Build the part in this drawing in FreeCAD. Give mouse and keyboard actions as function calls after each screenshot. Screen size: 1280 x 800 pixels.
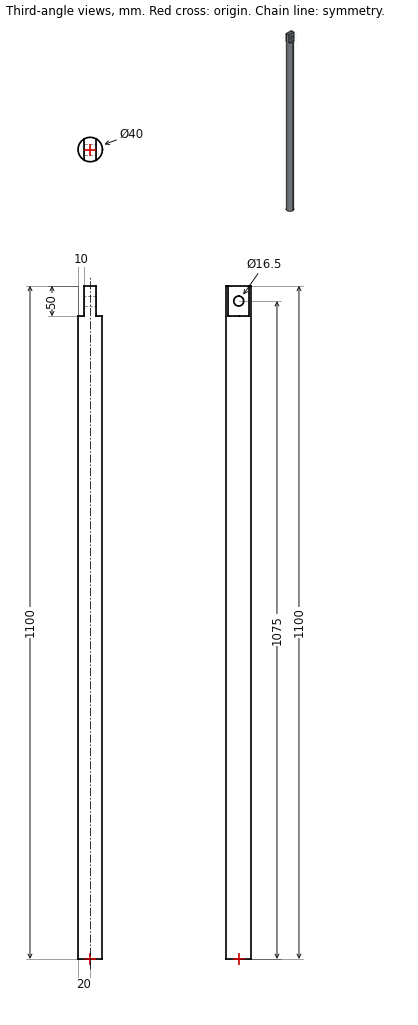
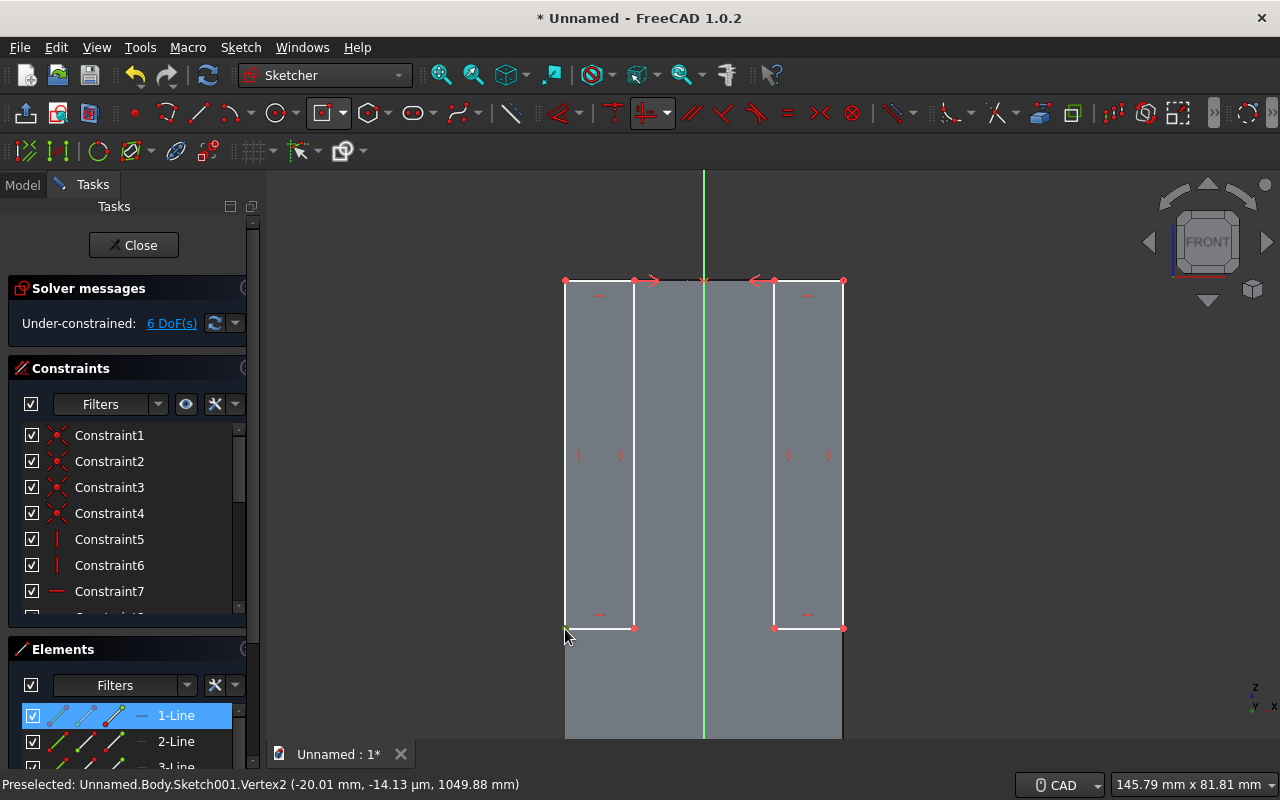
click(843, 629)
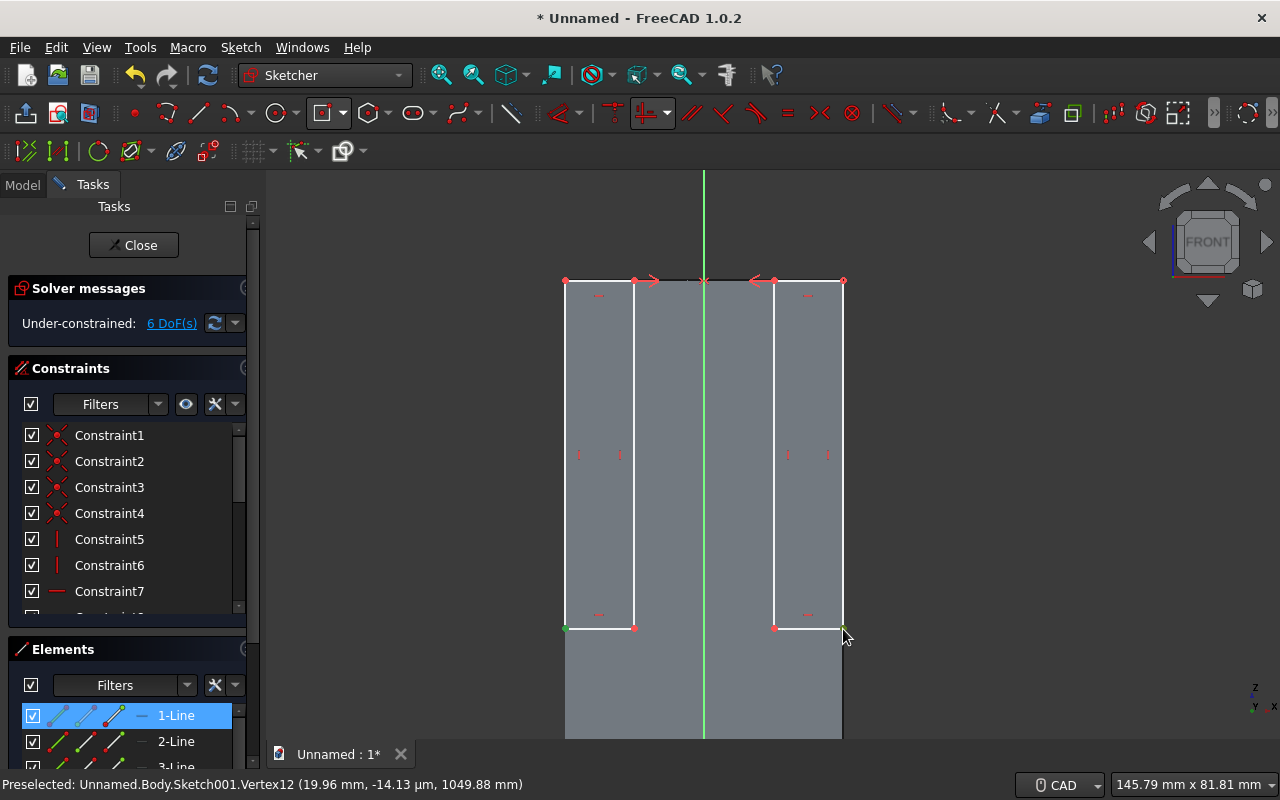
click(704, 674)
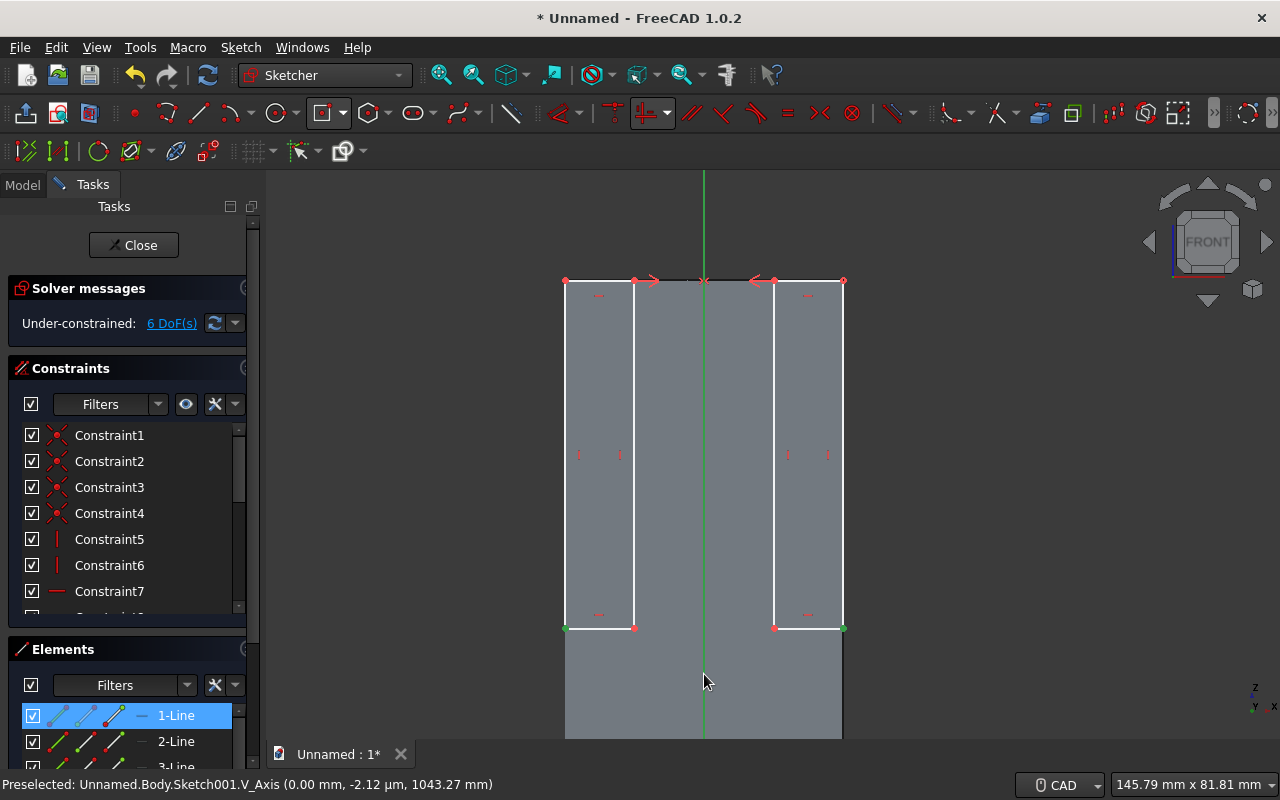
click(820, 114)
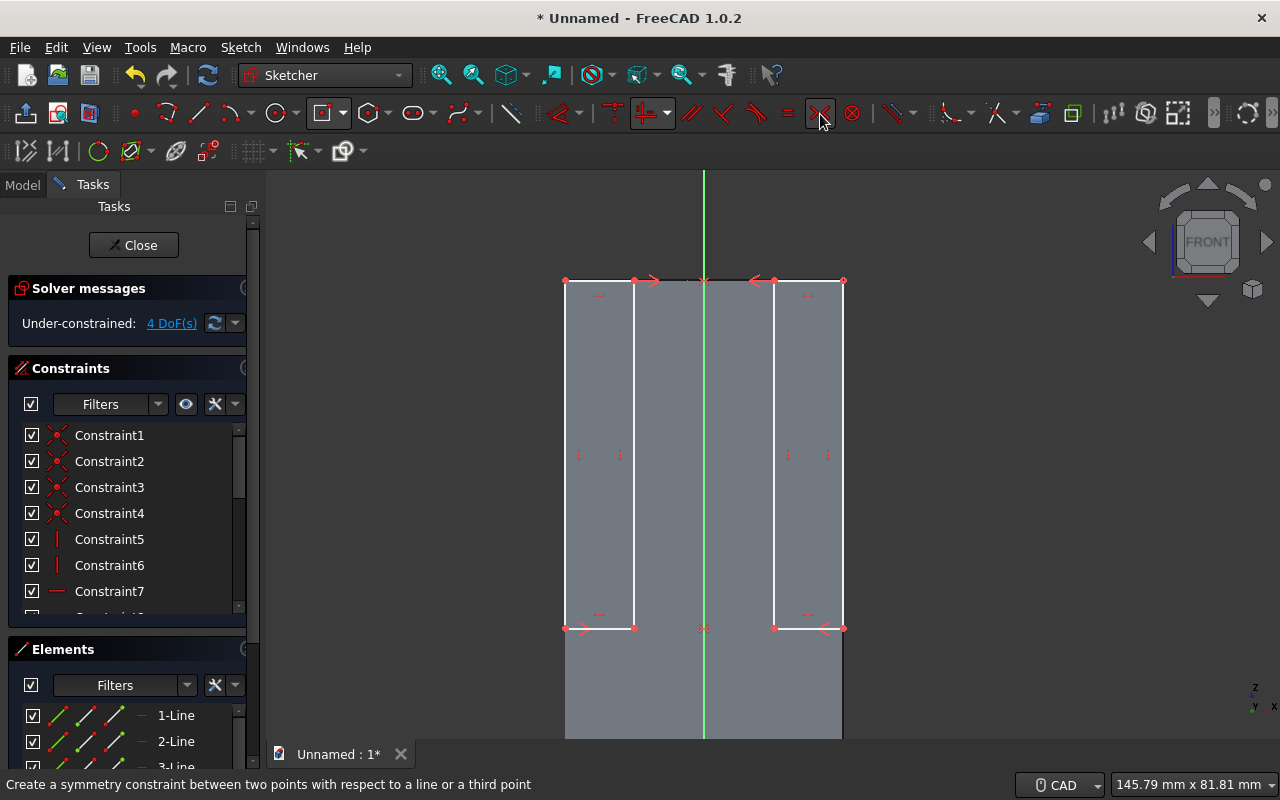
click(558, 114)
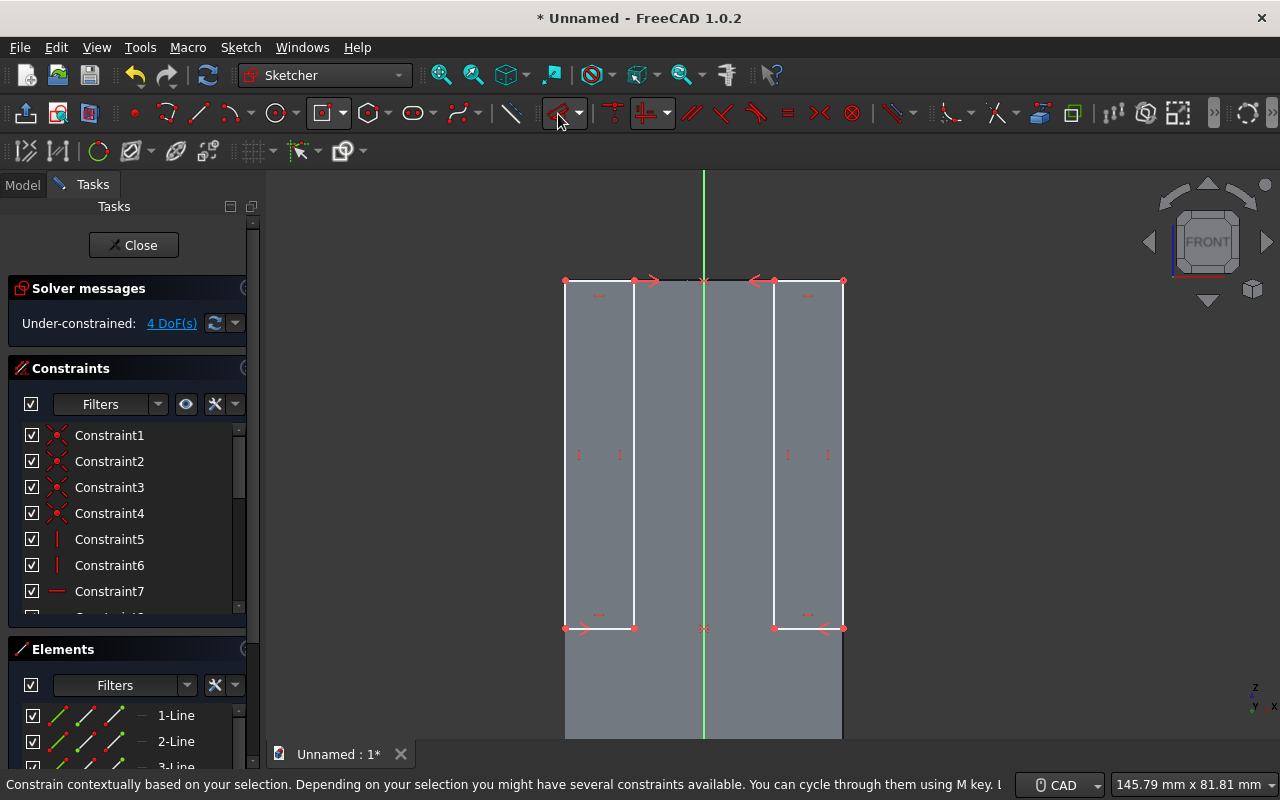
click(565, 385)
click(531, 455)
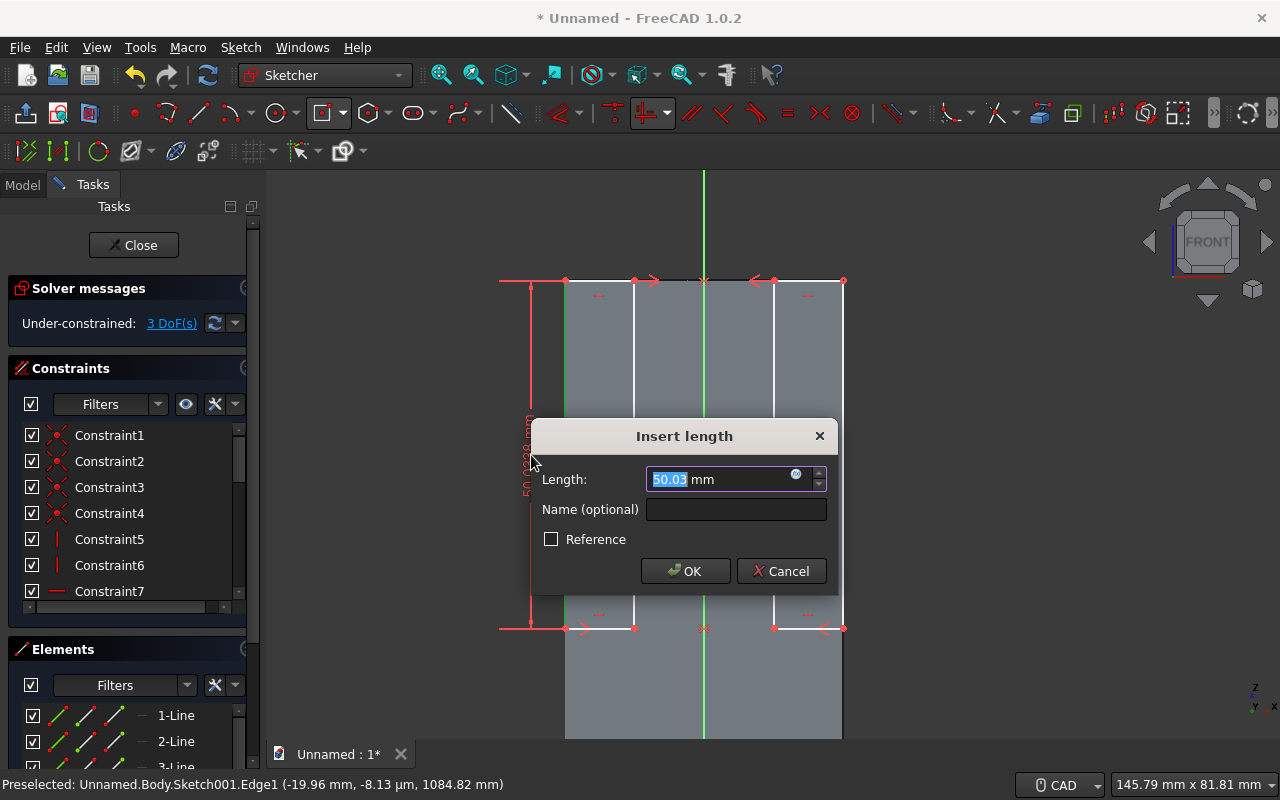
text(50)
key(Return)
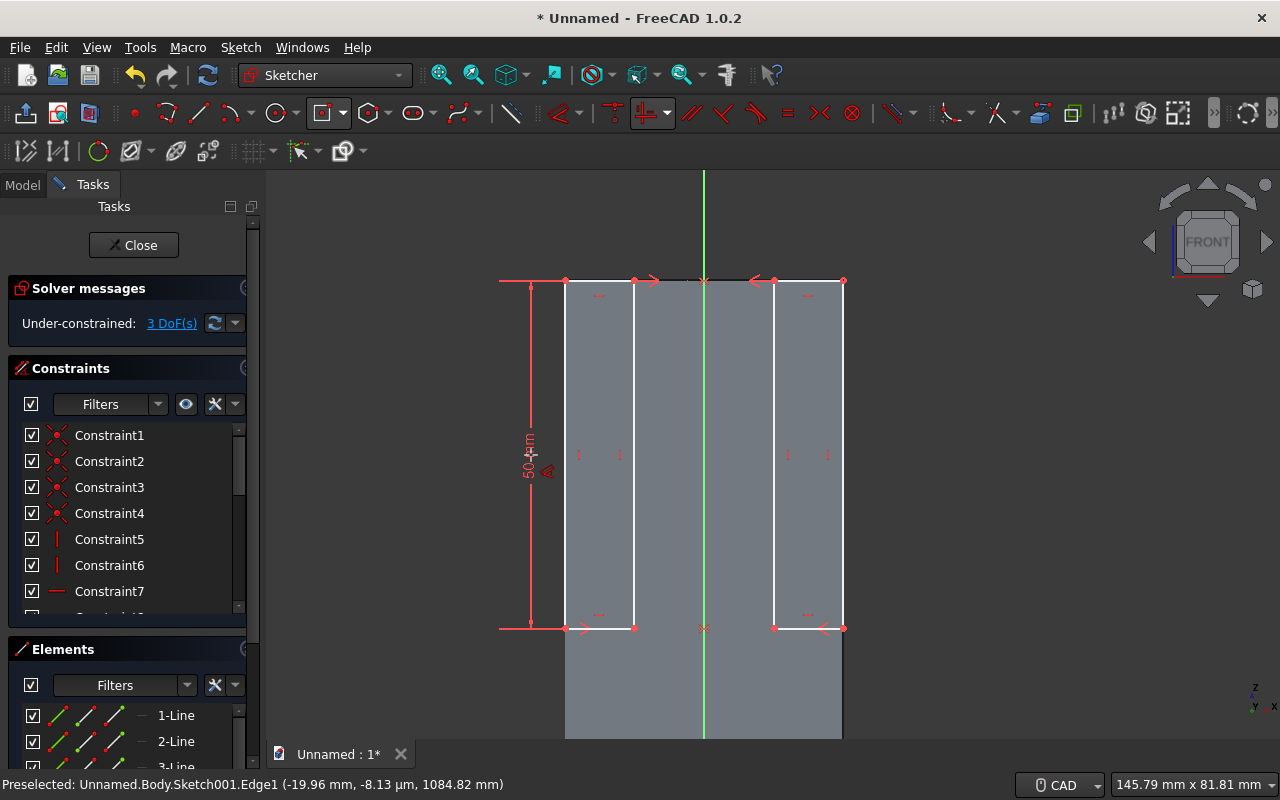
click(586, 629)
click(600, 663)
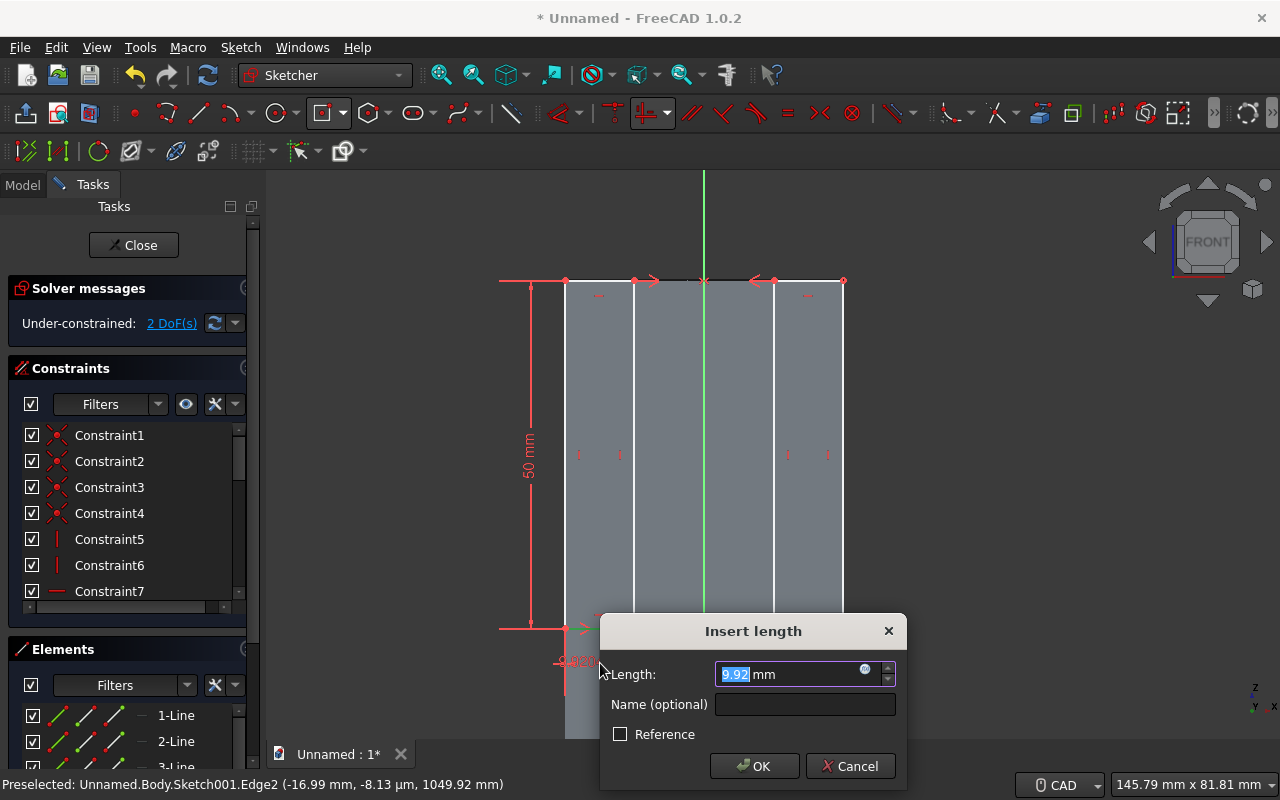
text(10)
key(Return)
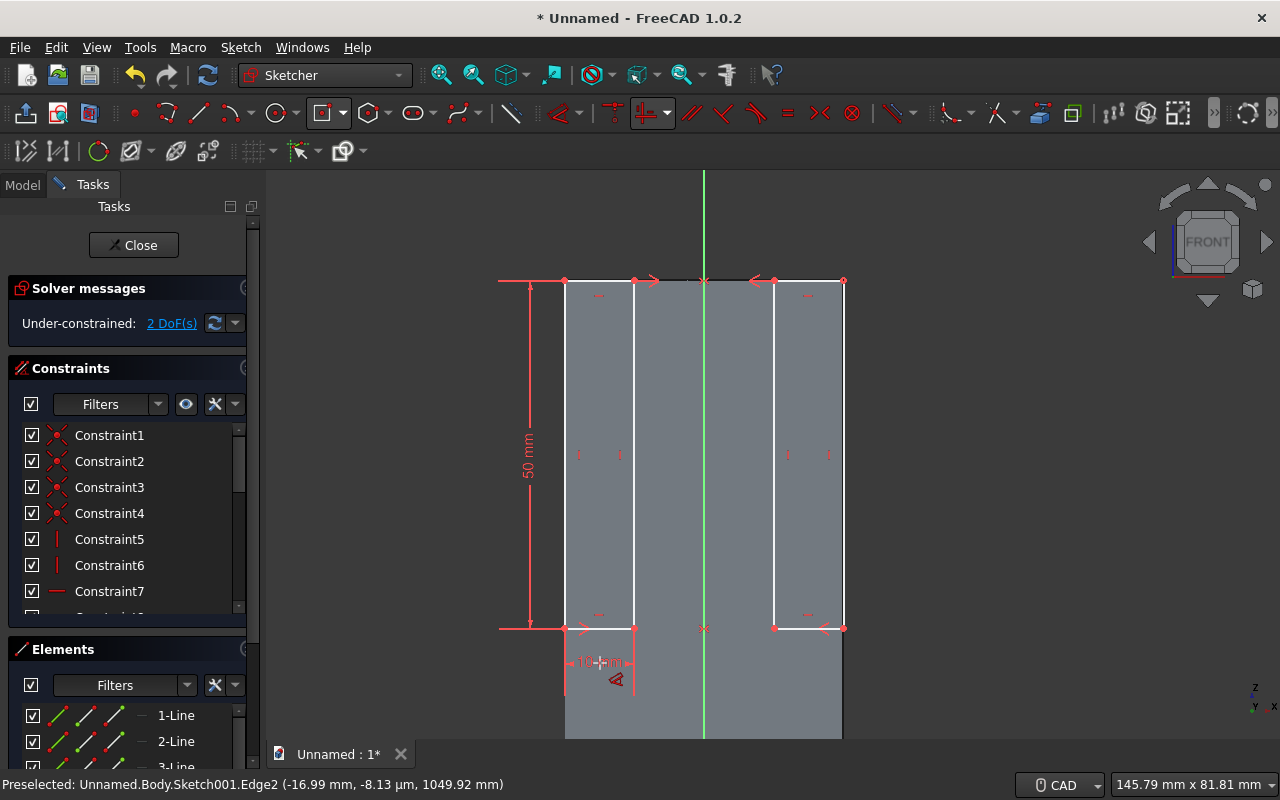
click(565, 281)
click(635, 247)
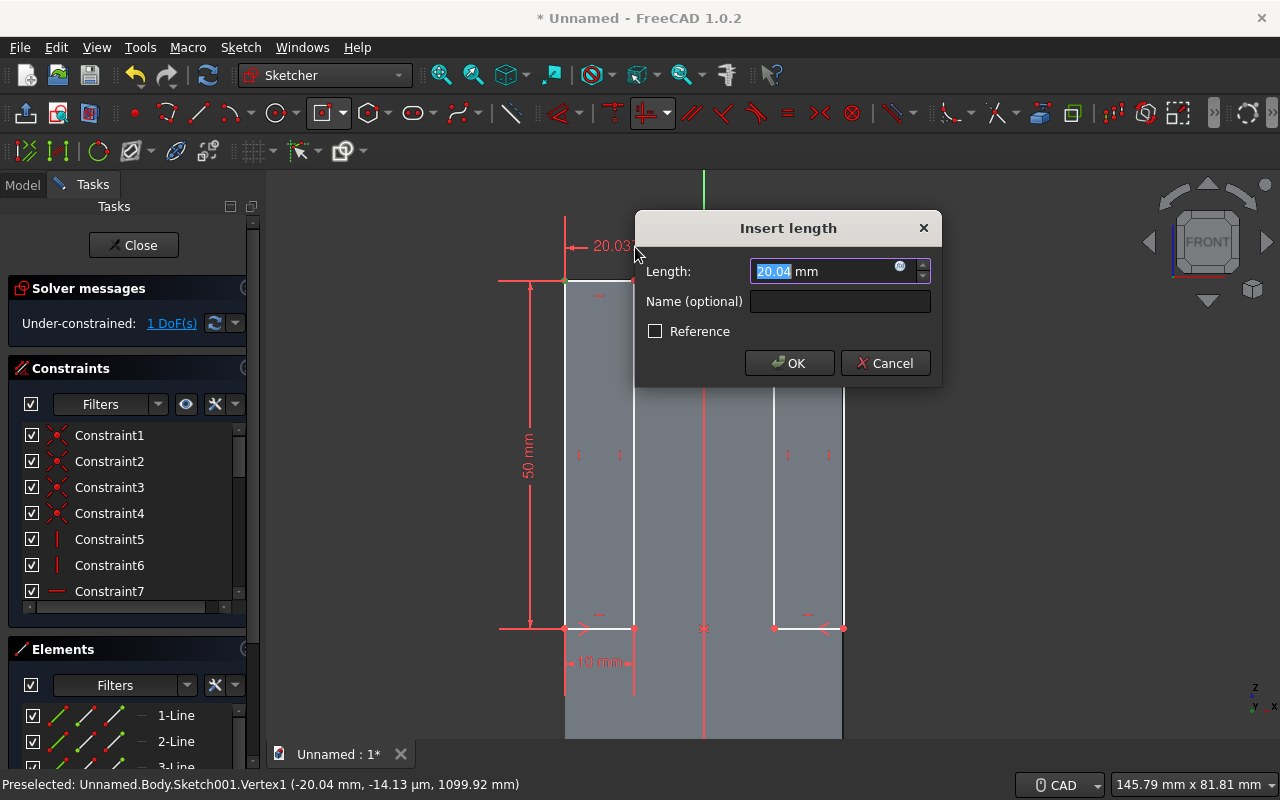
text(20)
key(Return)